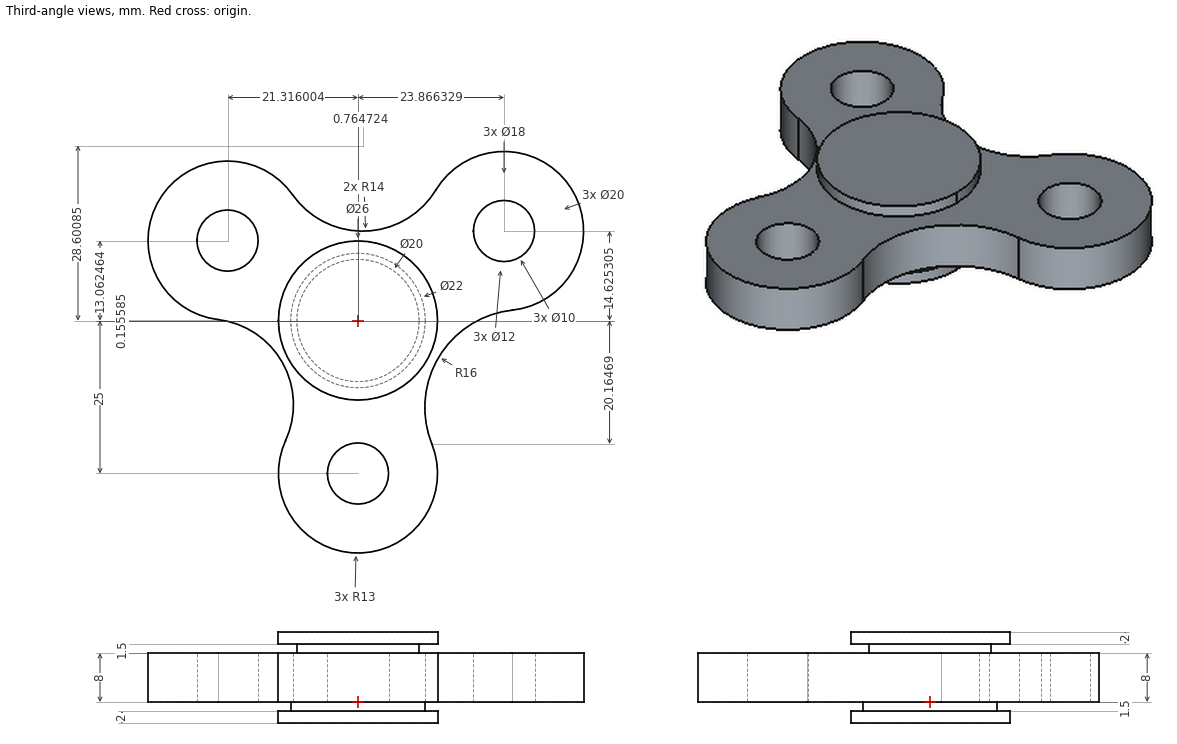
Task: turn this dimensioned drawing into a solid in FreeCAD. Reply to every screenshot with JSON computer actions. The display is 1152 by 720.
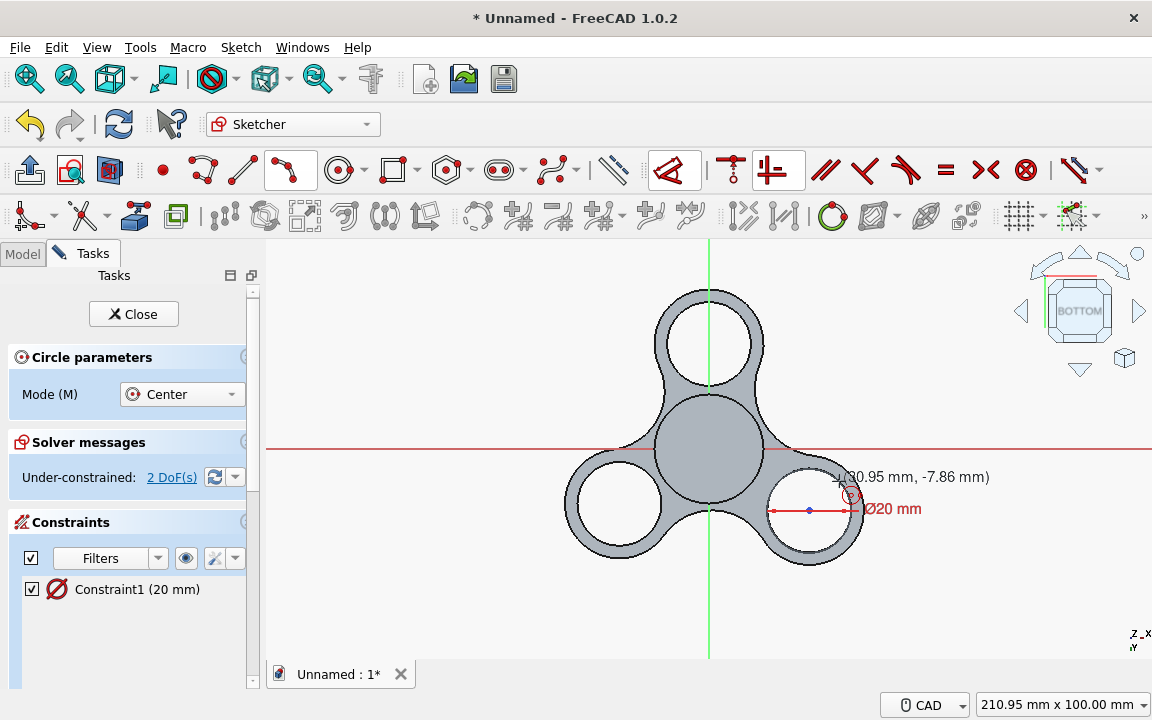
{"action": "left_click", "coordinate": [619, 504]}
{"action": "mouse_move", "coordinate": [649, 474]}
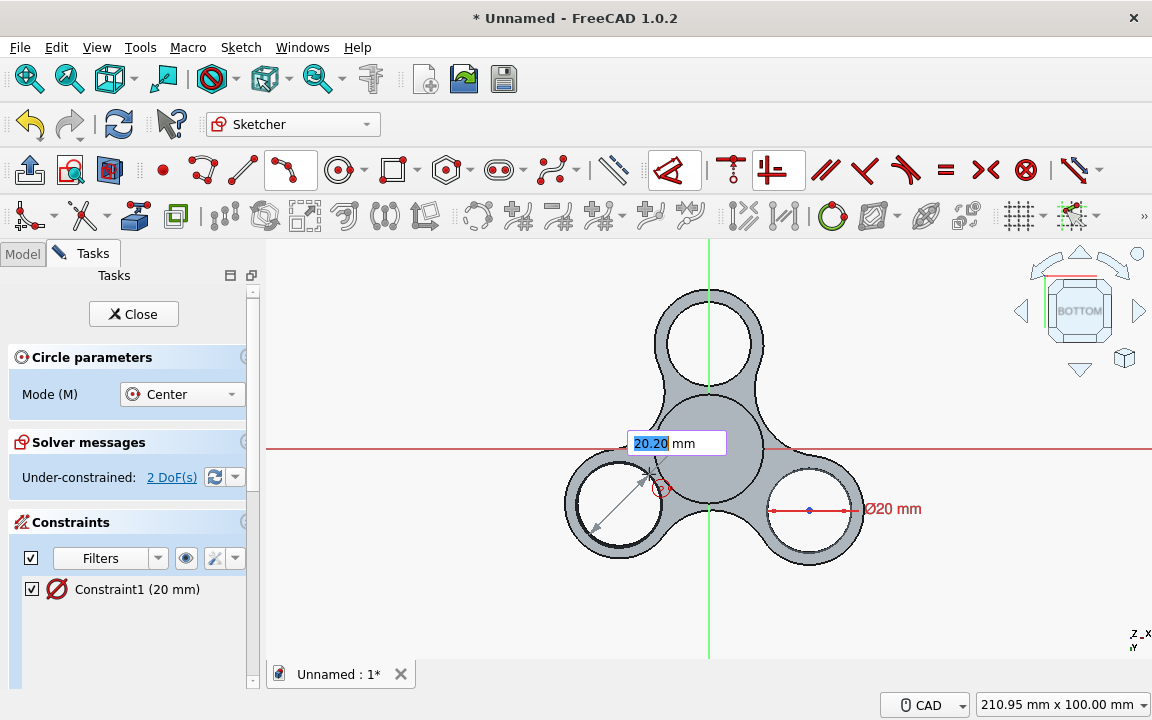
{"action": "type", "text": "20"}
{"action": "key", "text": "Return"}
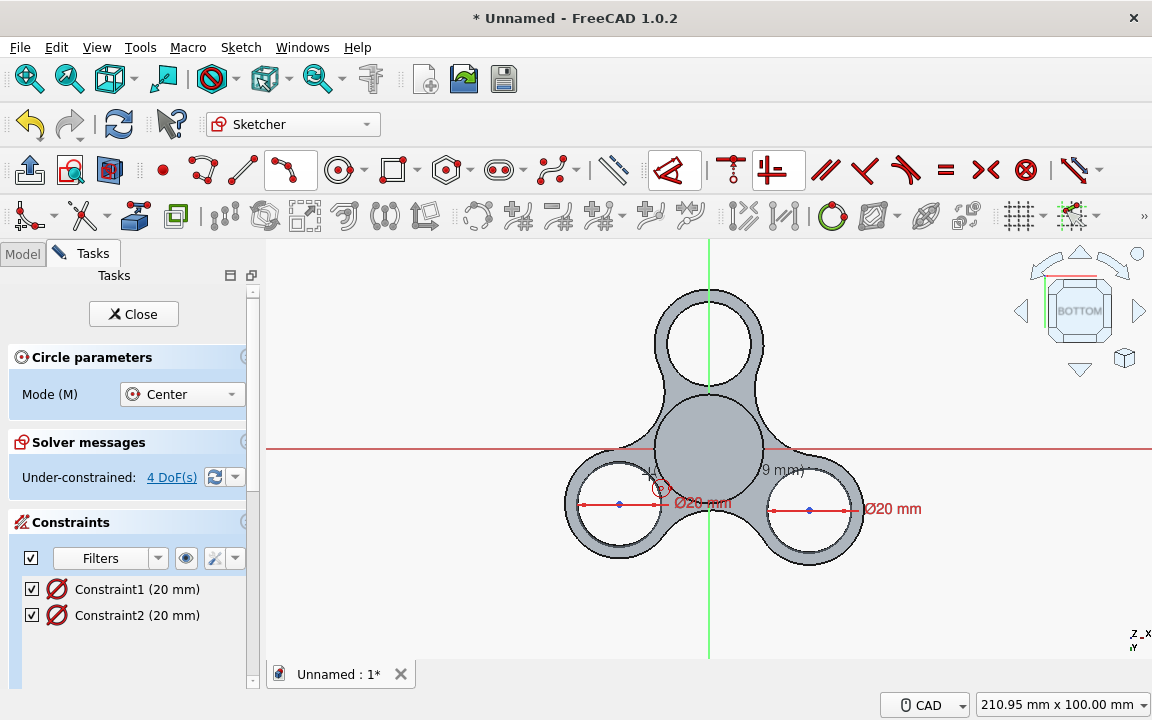
{"action": "left_click", "coordinate": [709, 344]}
{"action": "mouse_move", "coordinate": [739, 314]}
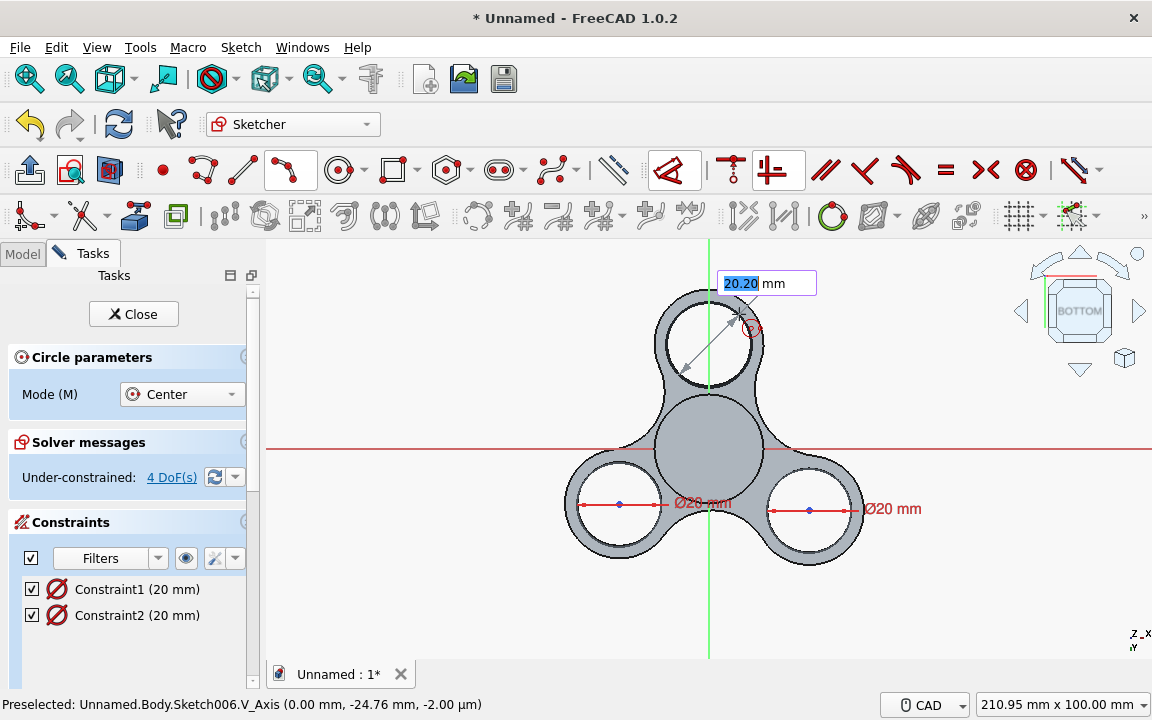
{"action": "type", "text": "20"}
{"action": "key", "text": "Return"}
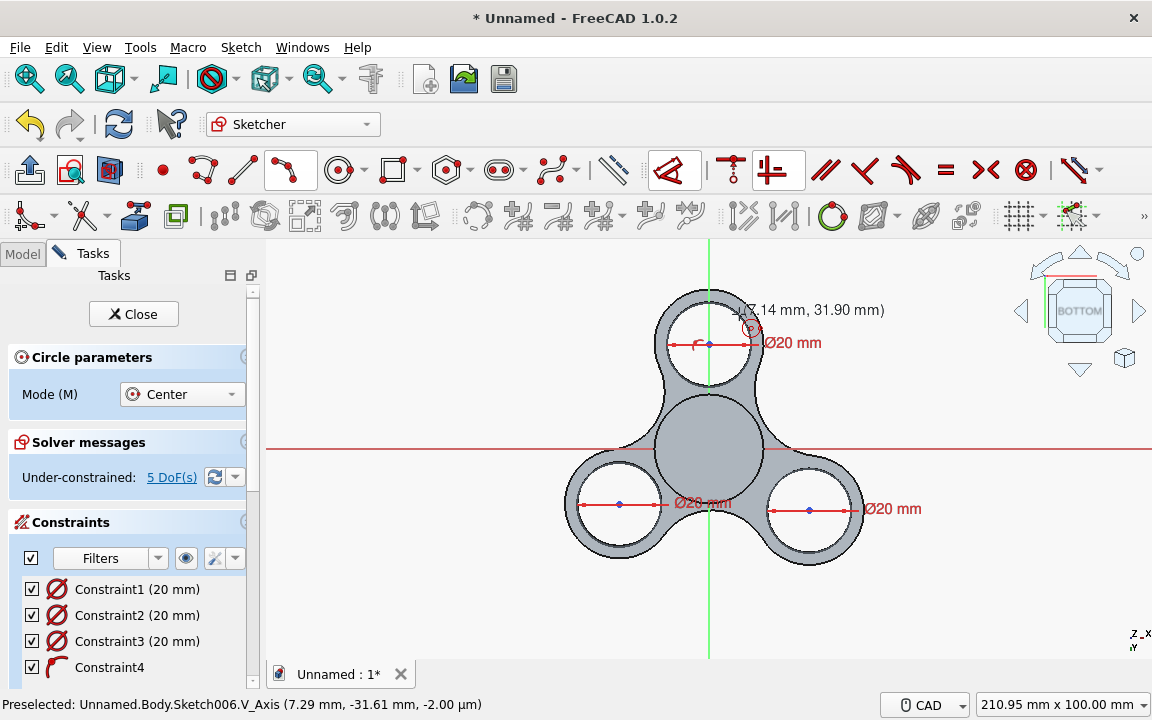
{"action": "left_click", "coordinate": [809, 511]}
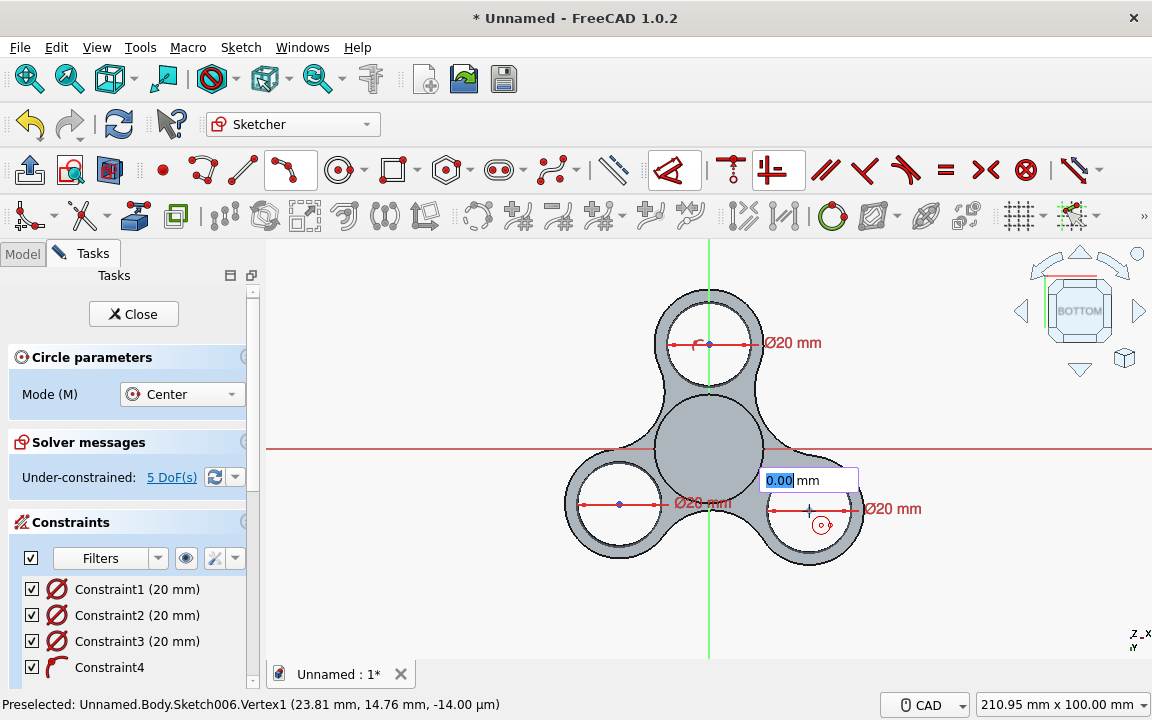
{"action": "scroll", "coordinate": [836, 537], "scroll_direction": "up", "scroll_amount": 7}
{"action": "mouse_move", "coordinate": [834, 535]}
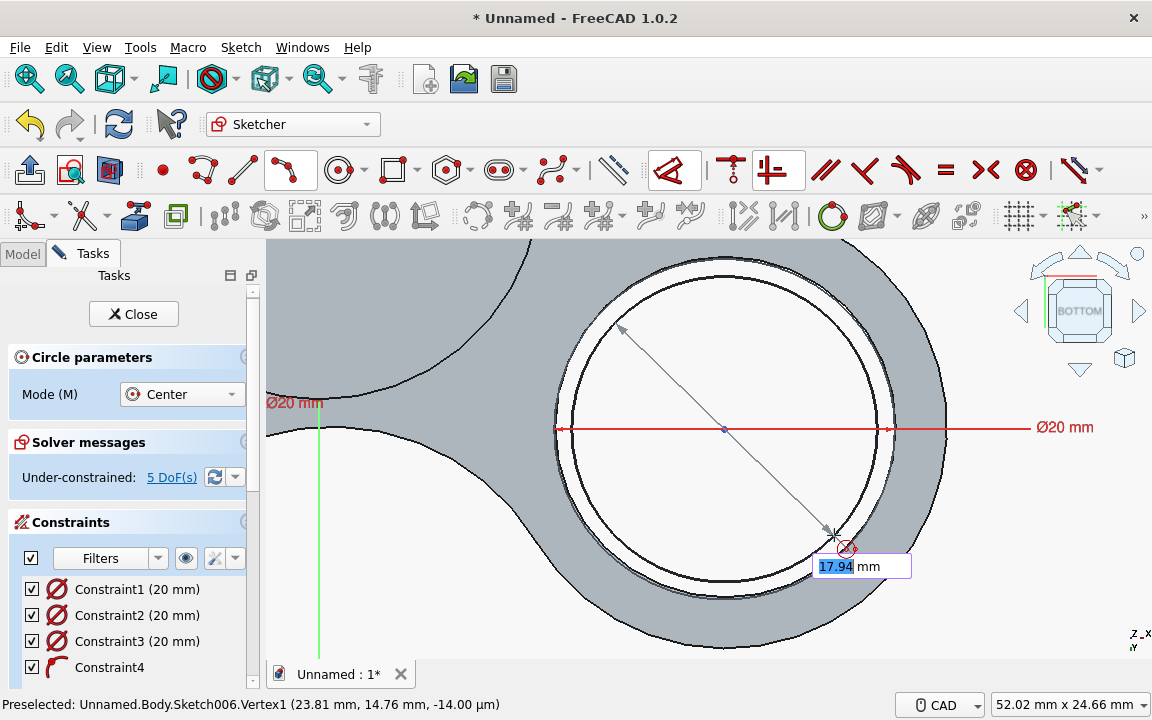
{"action": "type", "text": "18"}
{"action": "key", "text": "Return"}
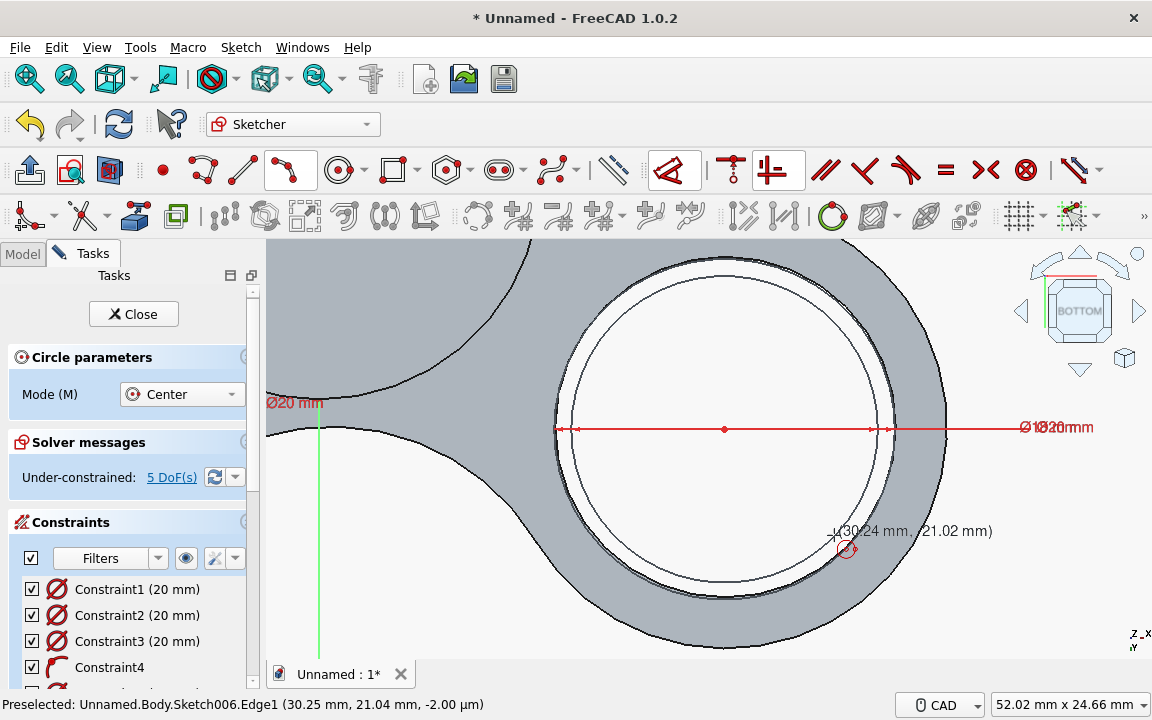
{"action": "scroll", "coordinate": [739, 567], "scroll_direction": "down", "scroll_amount": 7}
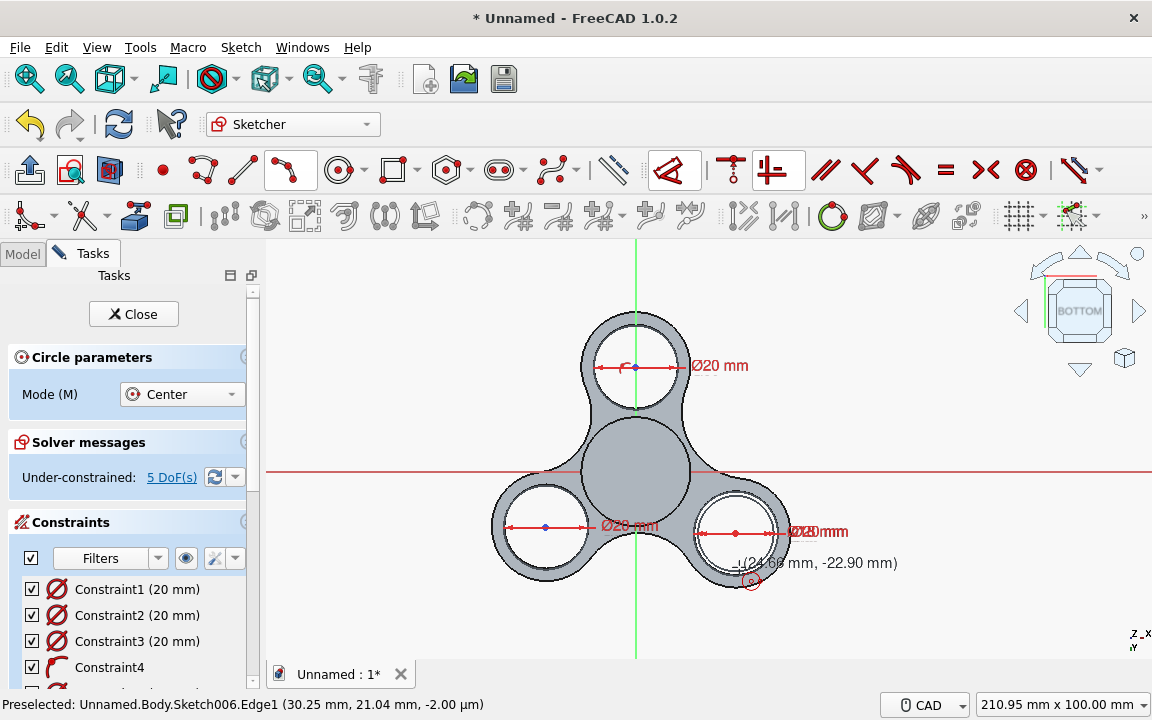
{"action": "left_click", "coordinate": [546, 528]}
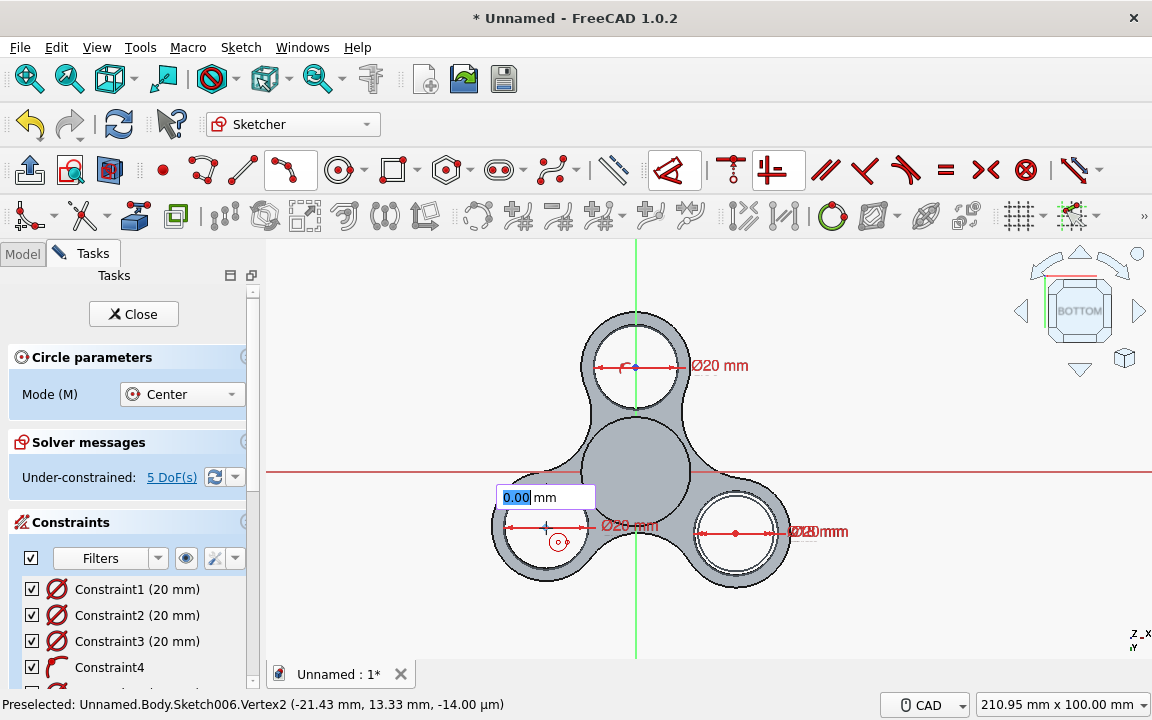
{"action": "scroll", "coordinate": [511, 514], "scroll_direction": "up", "scroll_amount": 7}
{"action": "mouse_move", "coordinate": [509, 510]}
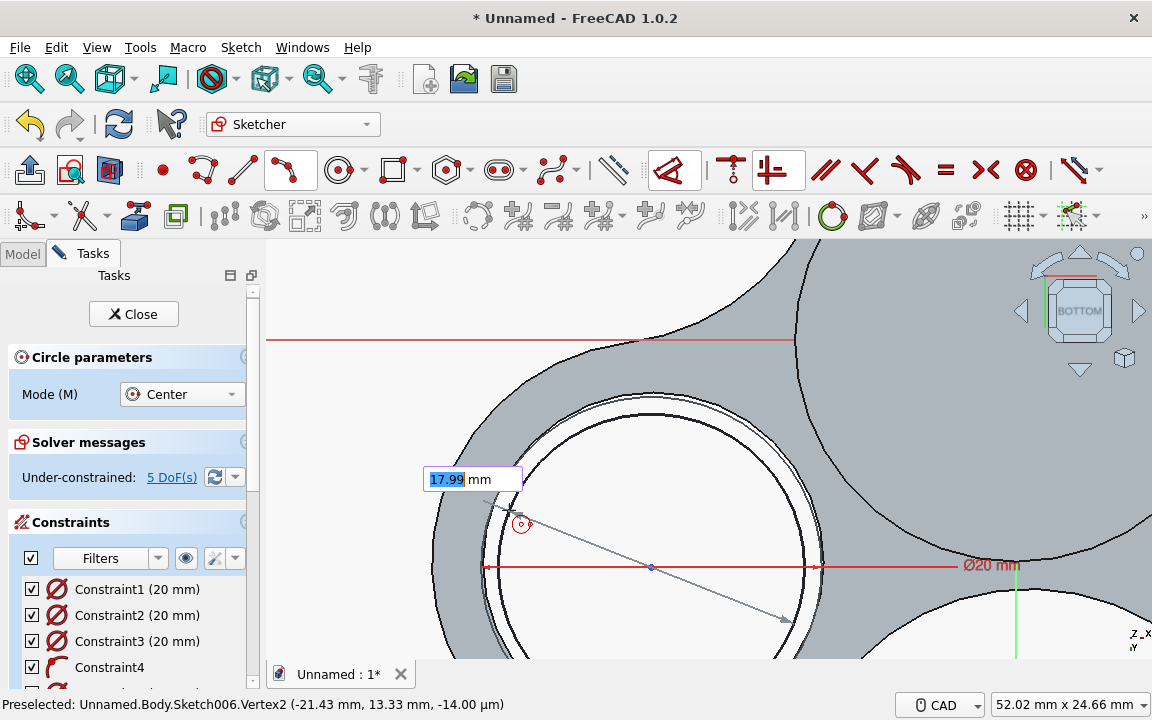
{"action": "type", "text": "18"}
{"action": "key", "text": "Return"}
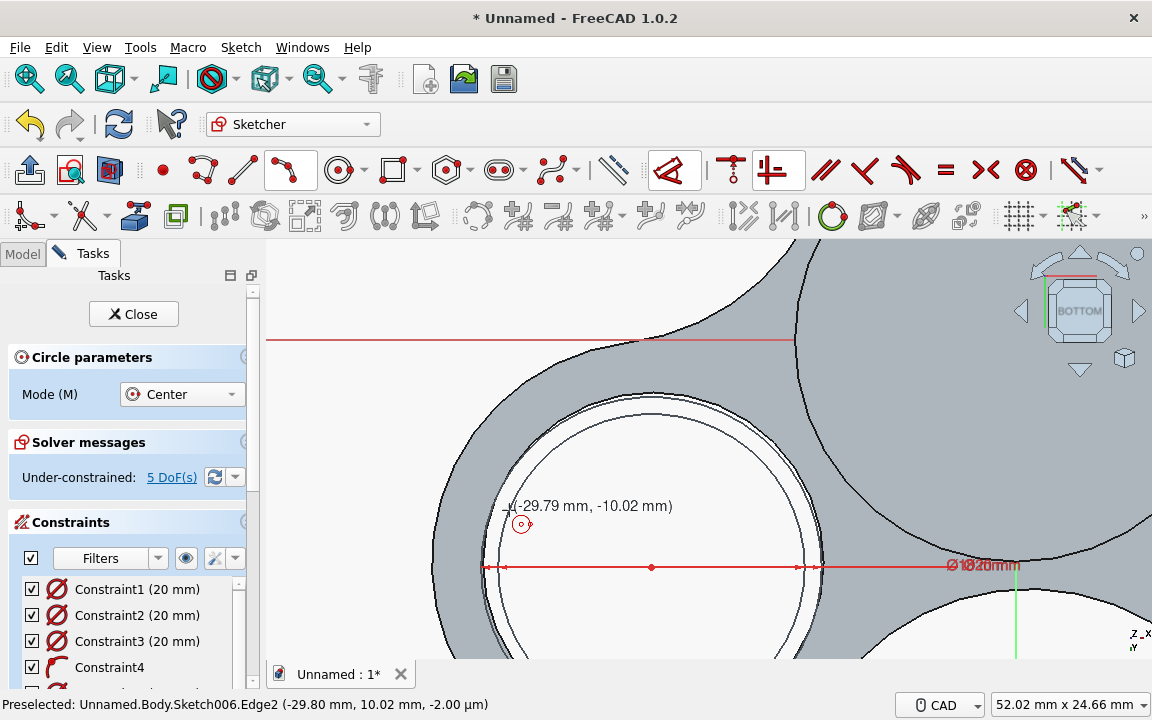
{"action": "scroll", "coordinate": [510, 514], "scroll_direction": "down", "scroll_amount": 7}